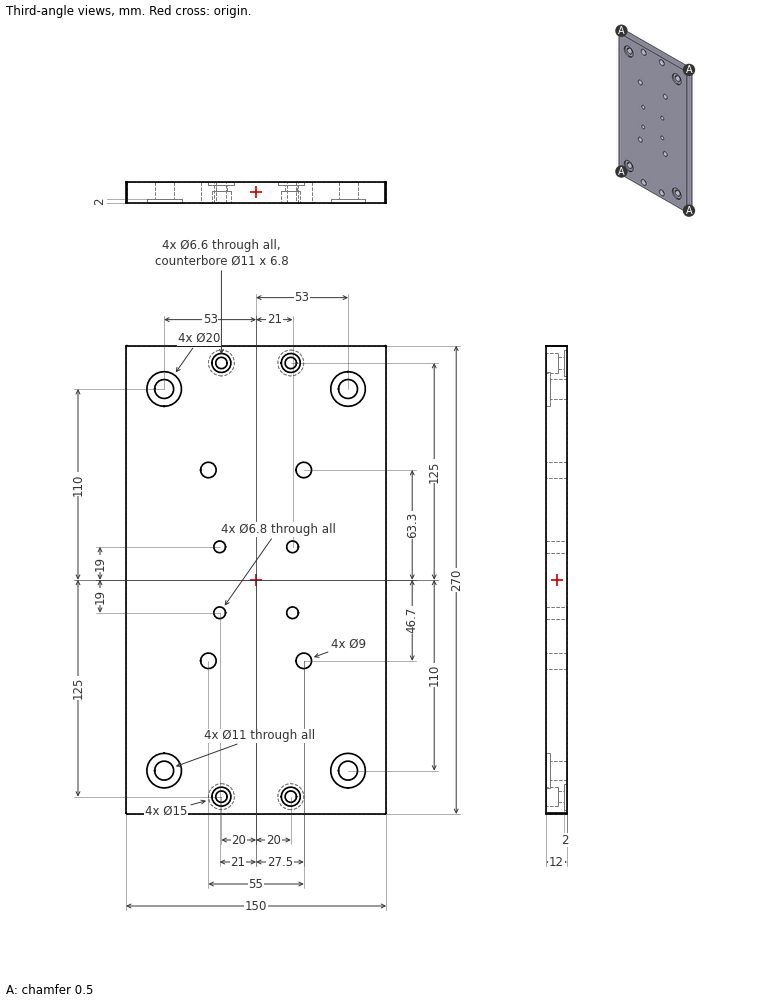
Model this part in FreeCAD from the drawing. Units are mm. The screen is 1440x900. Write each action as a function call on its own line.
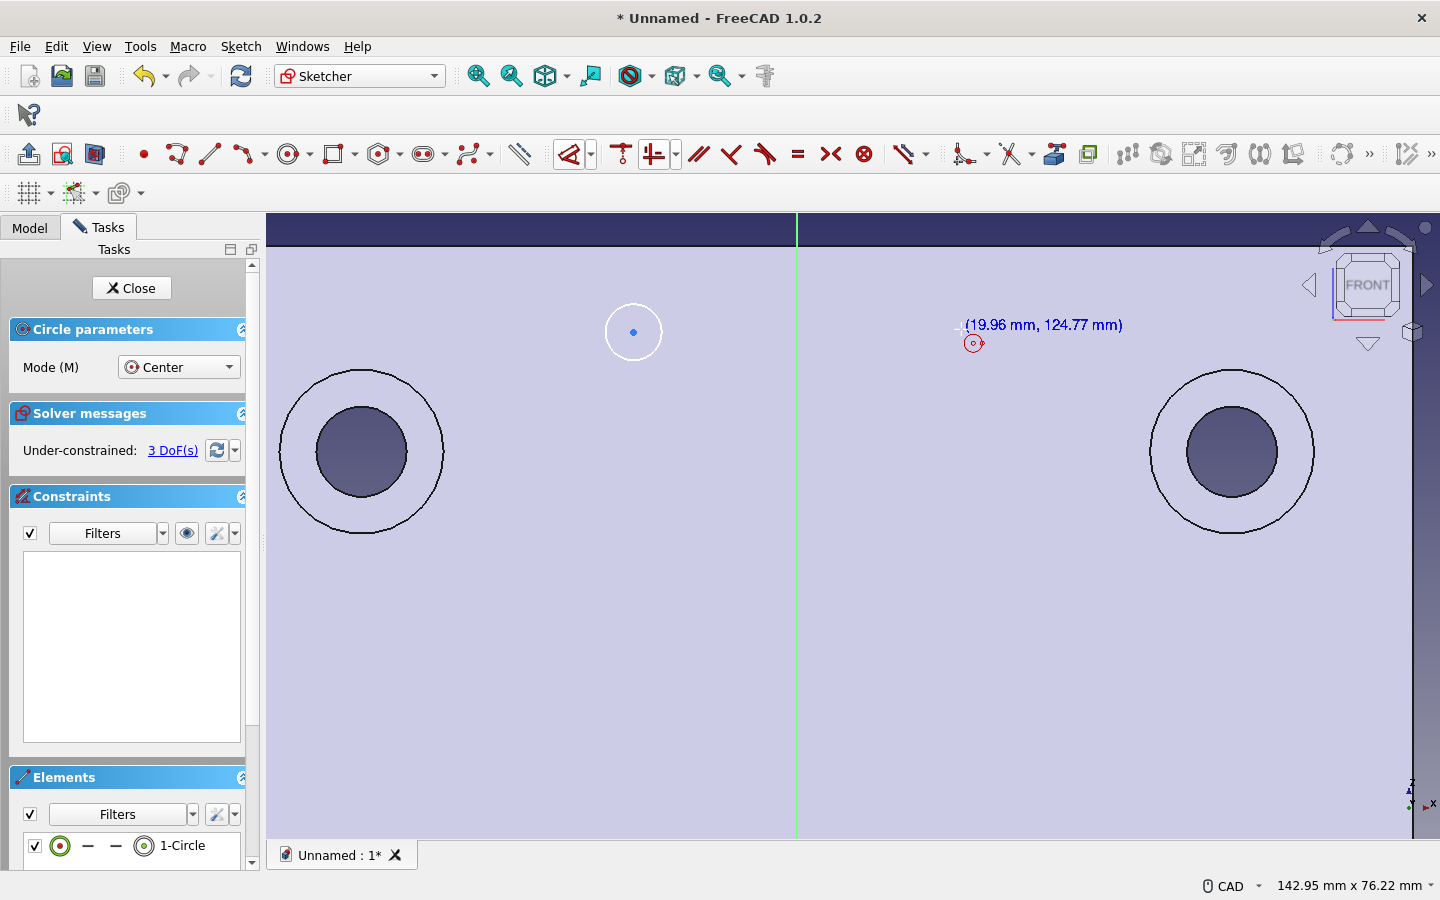
scroll(781, 316, down, 8)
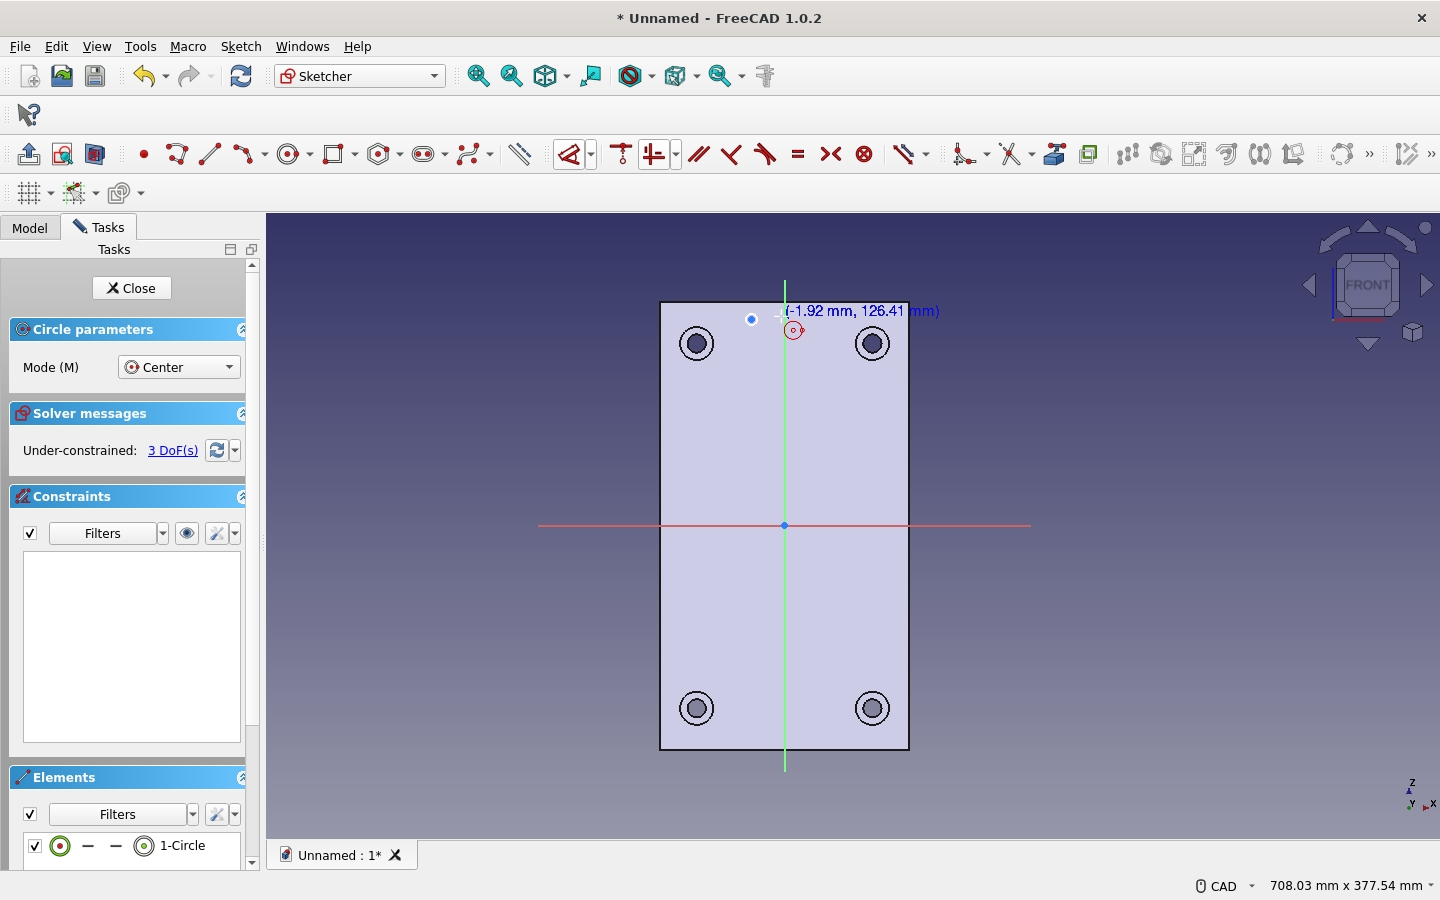
click(818, 319)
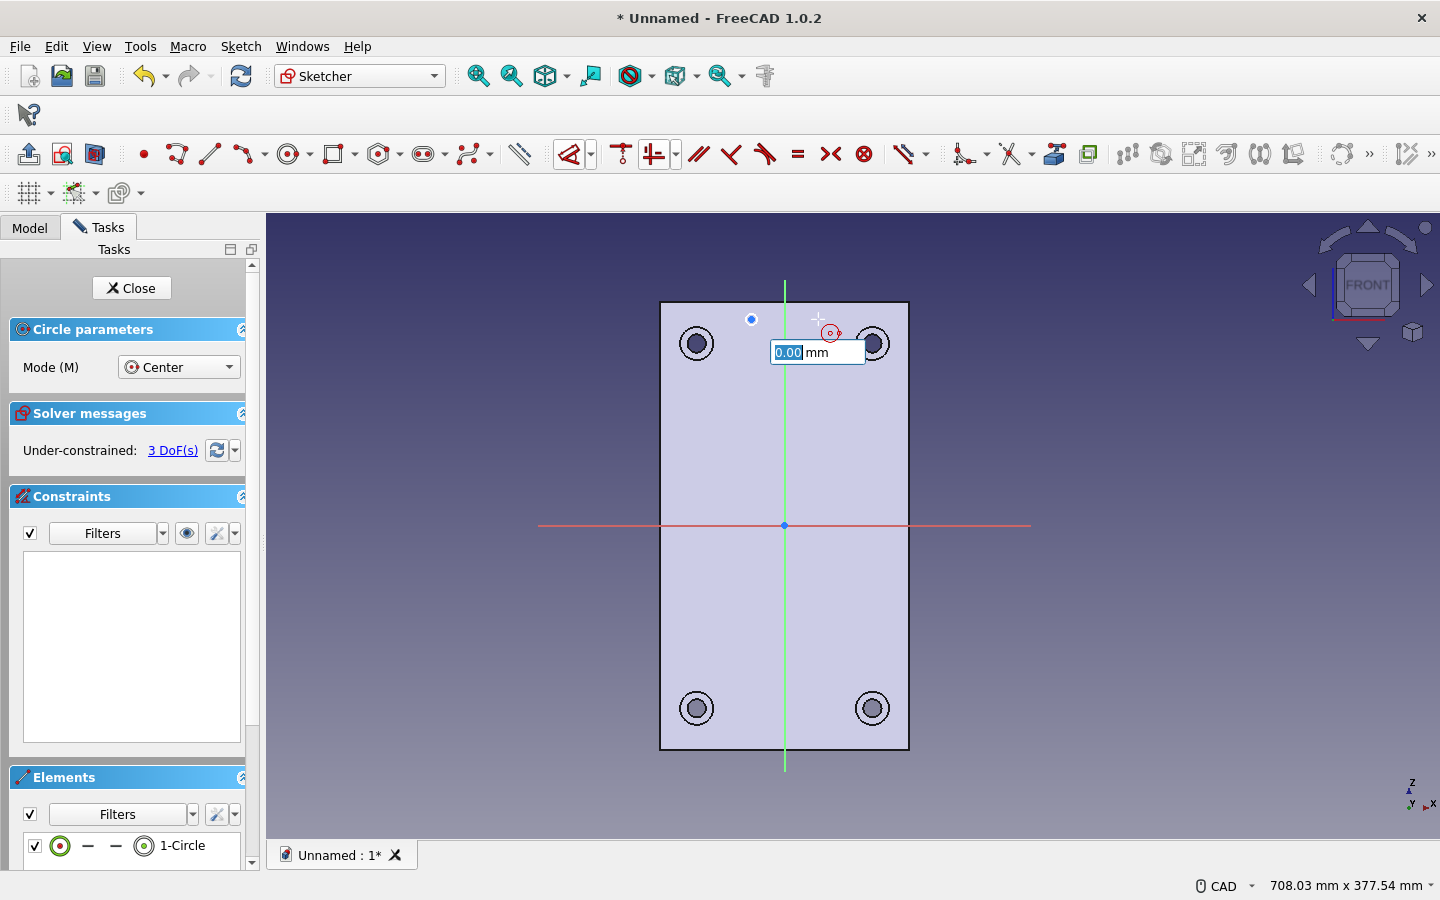
scroll(822, 315, up, 6)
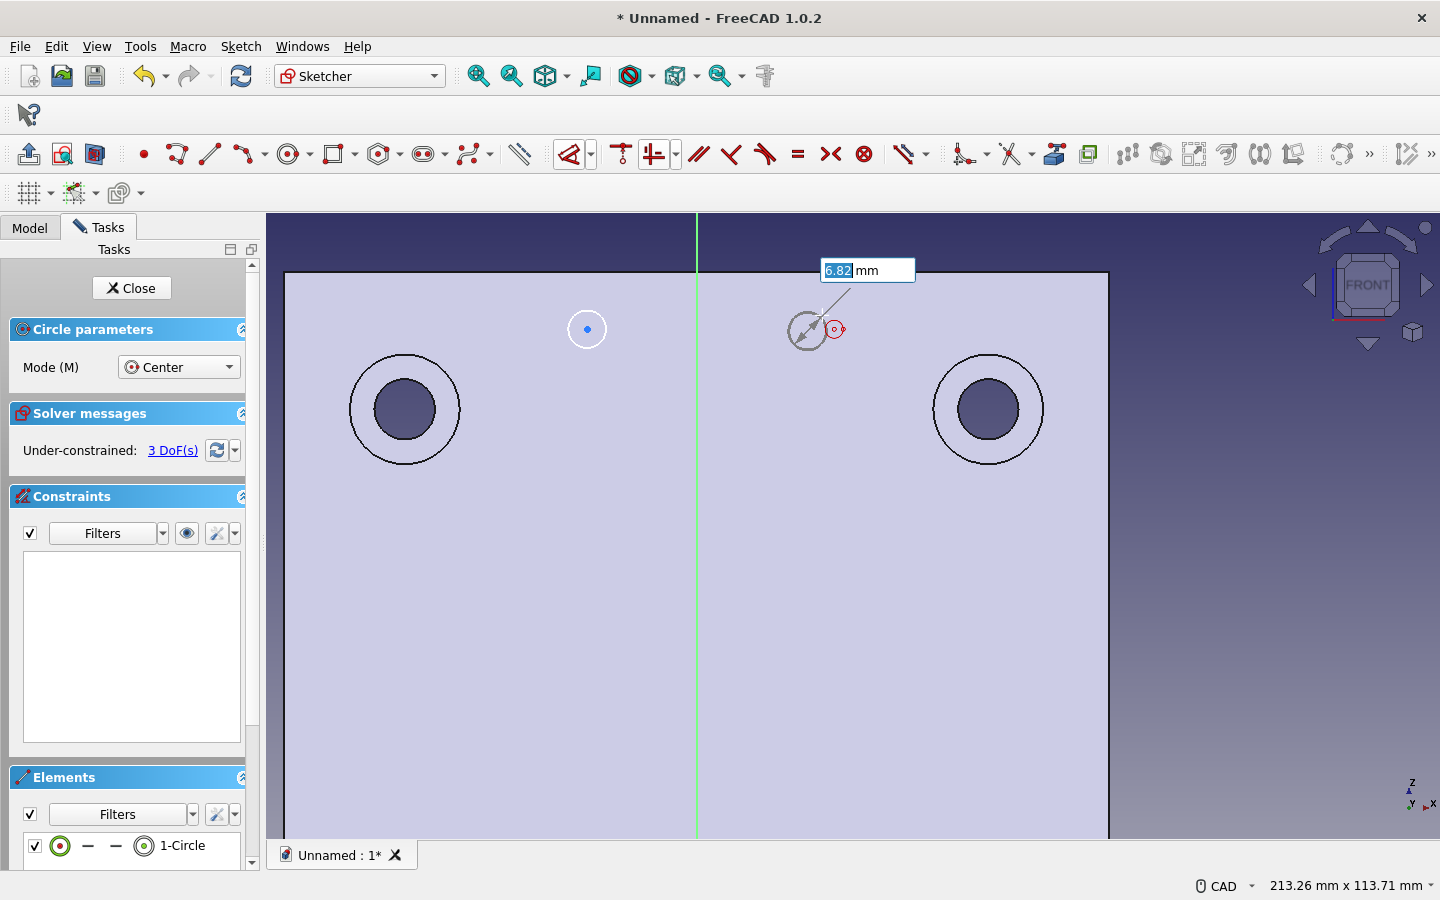
click(819, 314)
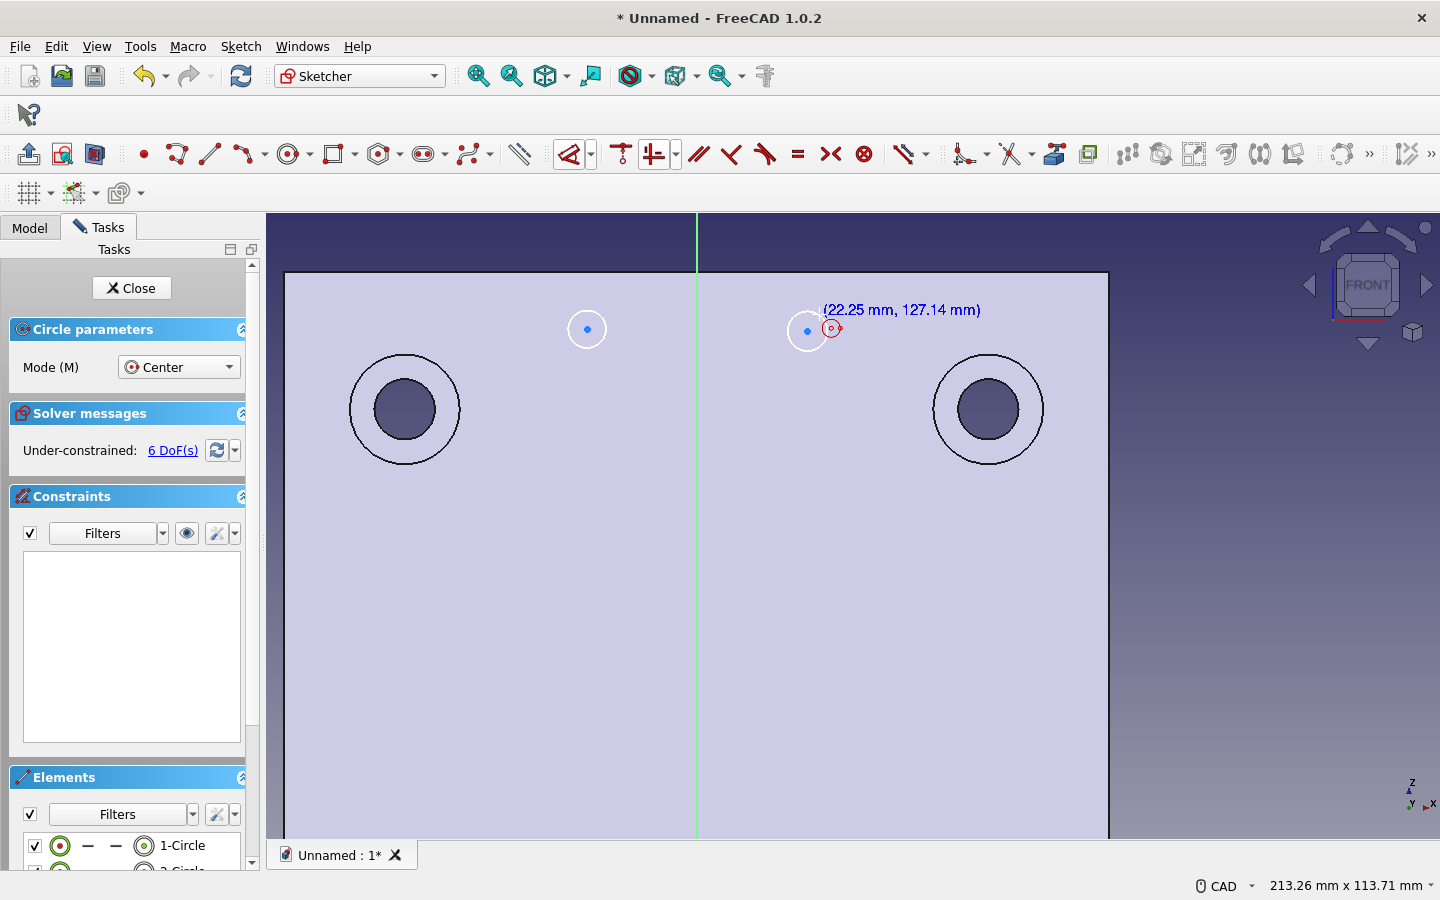
scroll(822, 315, down, 6)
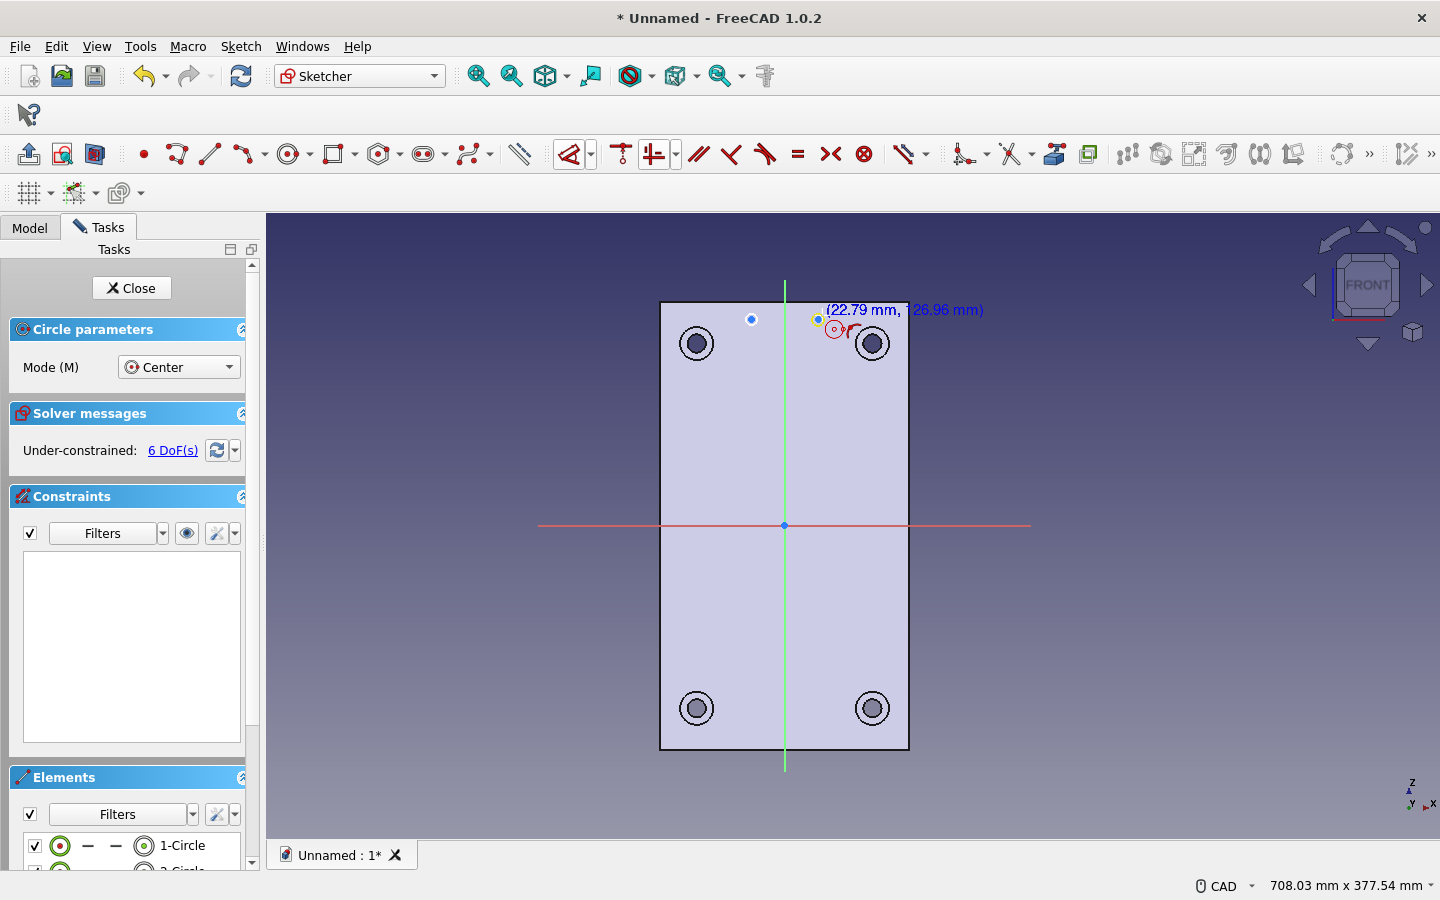
scroll(751, 733, up, 8)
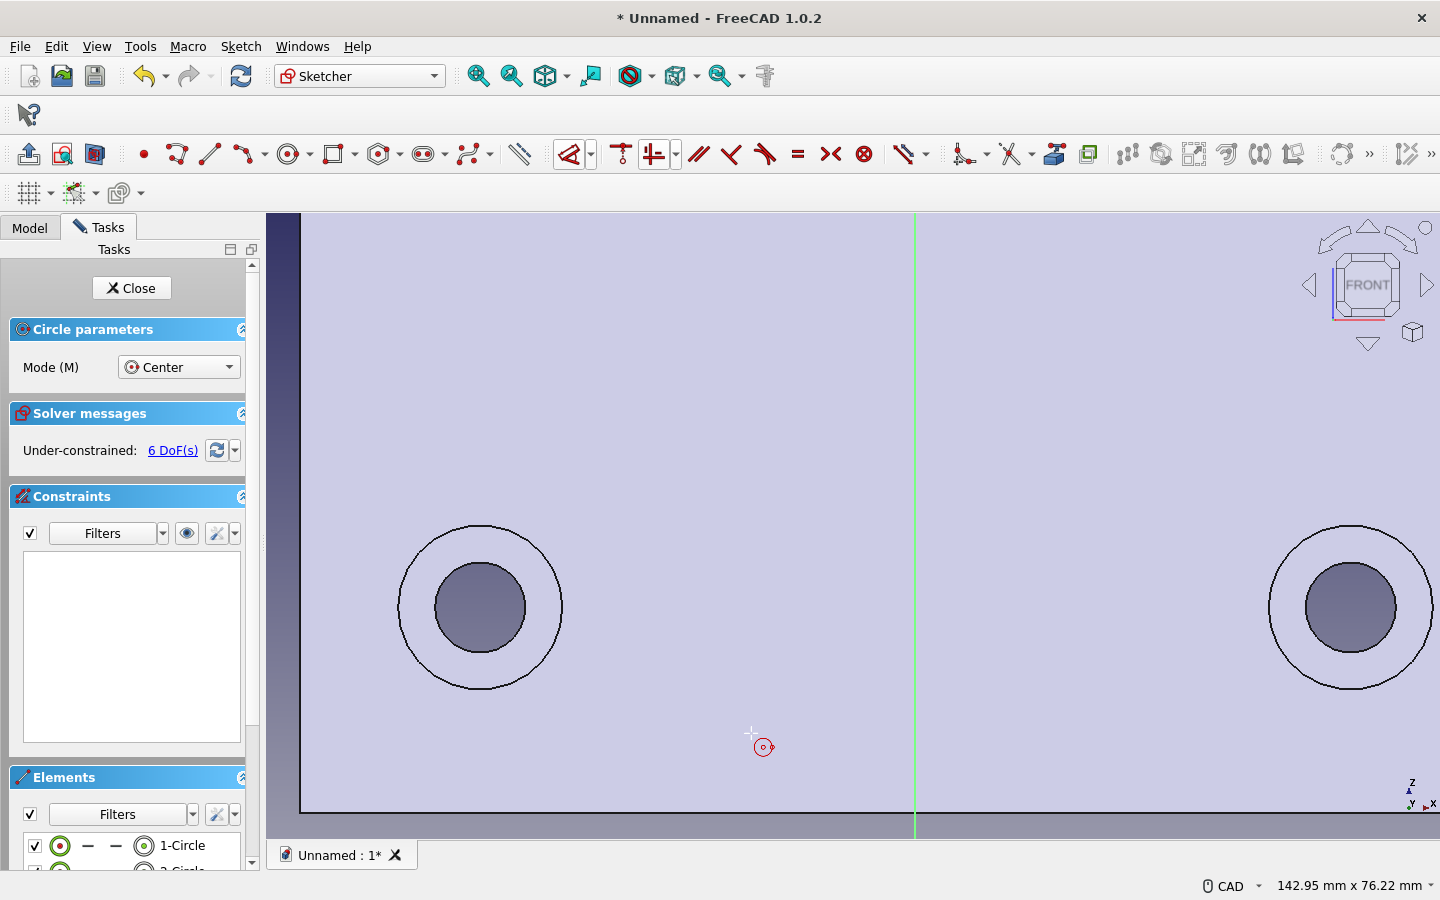
scroll(751, 734, down, 8)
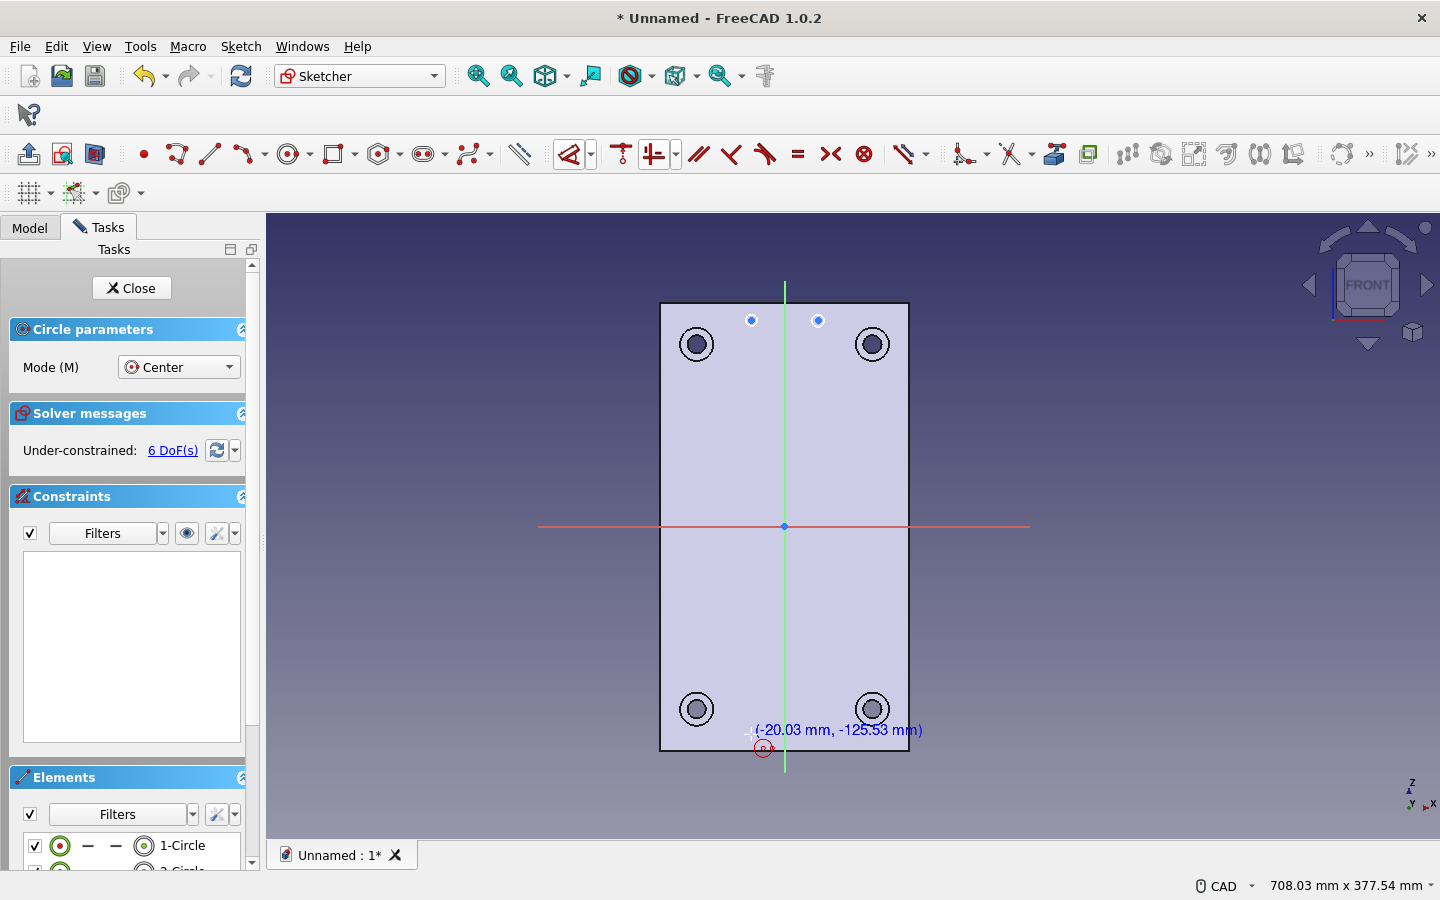
click(751, 734)